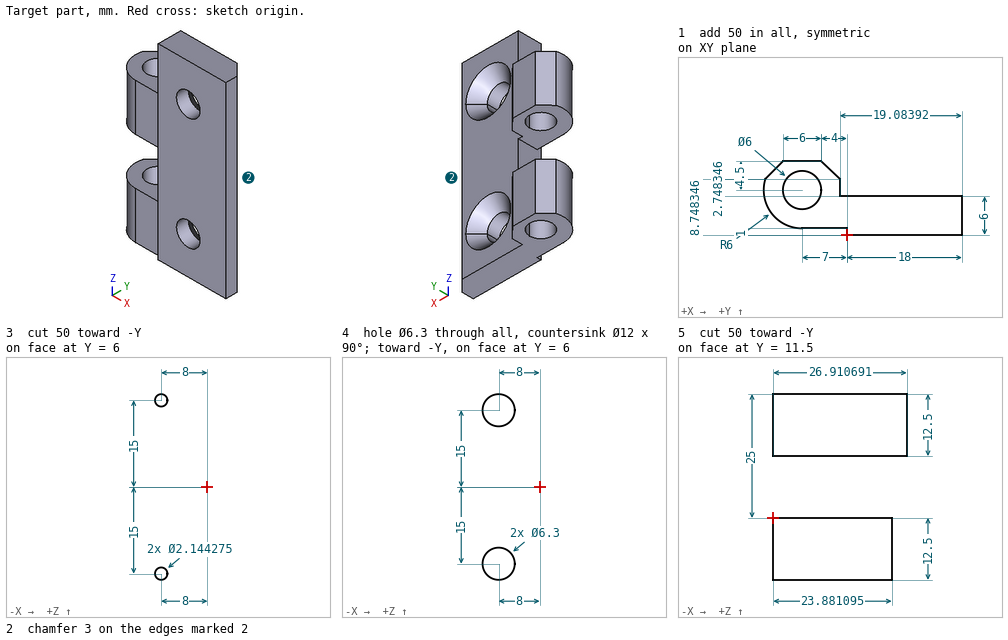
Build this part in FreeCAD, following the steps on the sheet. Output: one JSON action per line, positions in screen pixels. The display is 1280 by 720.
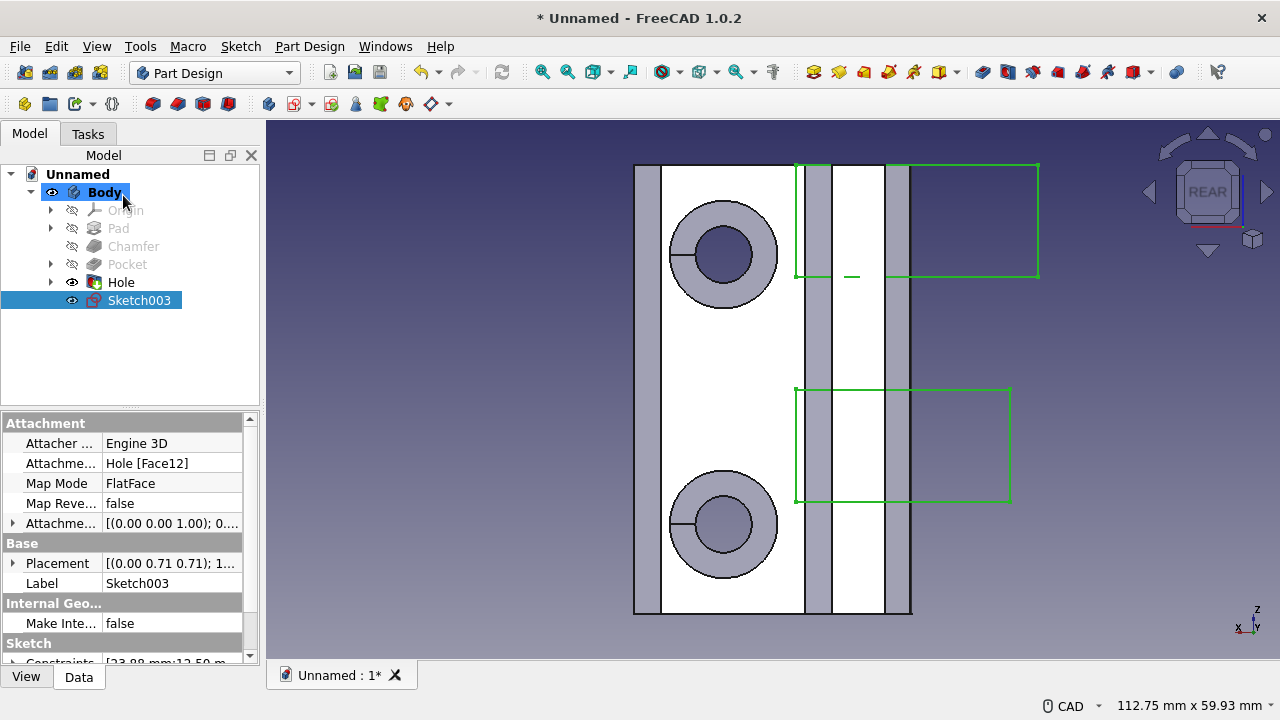
{"action": "left_click", "coordinate": [983, 72]}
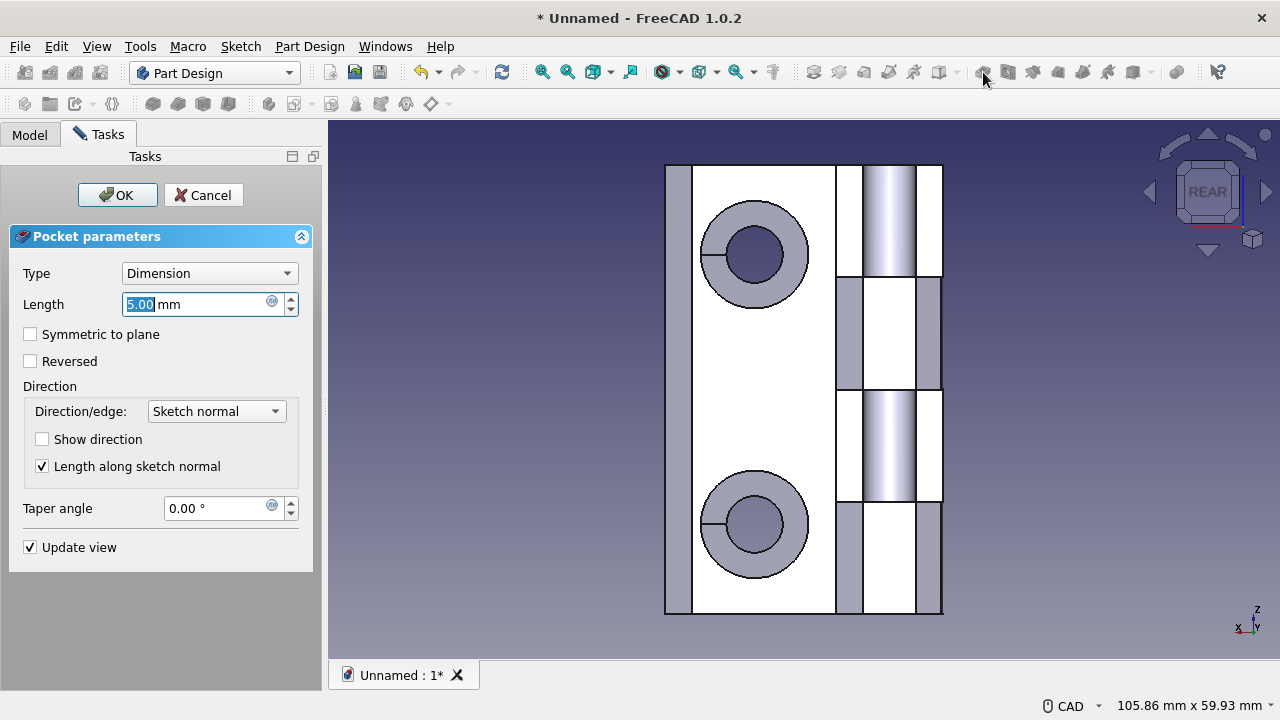
{"action": "type", "text": "50"}
{"action": "key", "text": "Tab"}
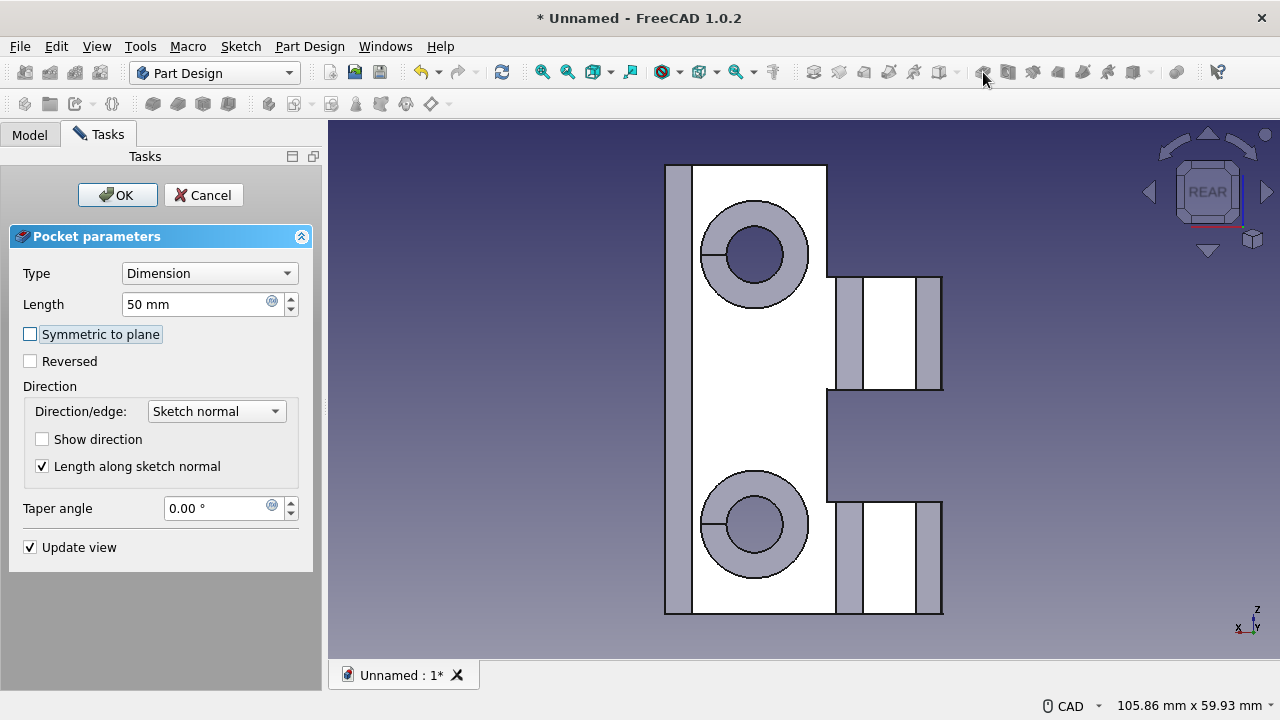
{"action": "left_click", "coordinate": [118, 195]}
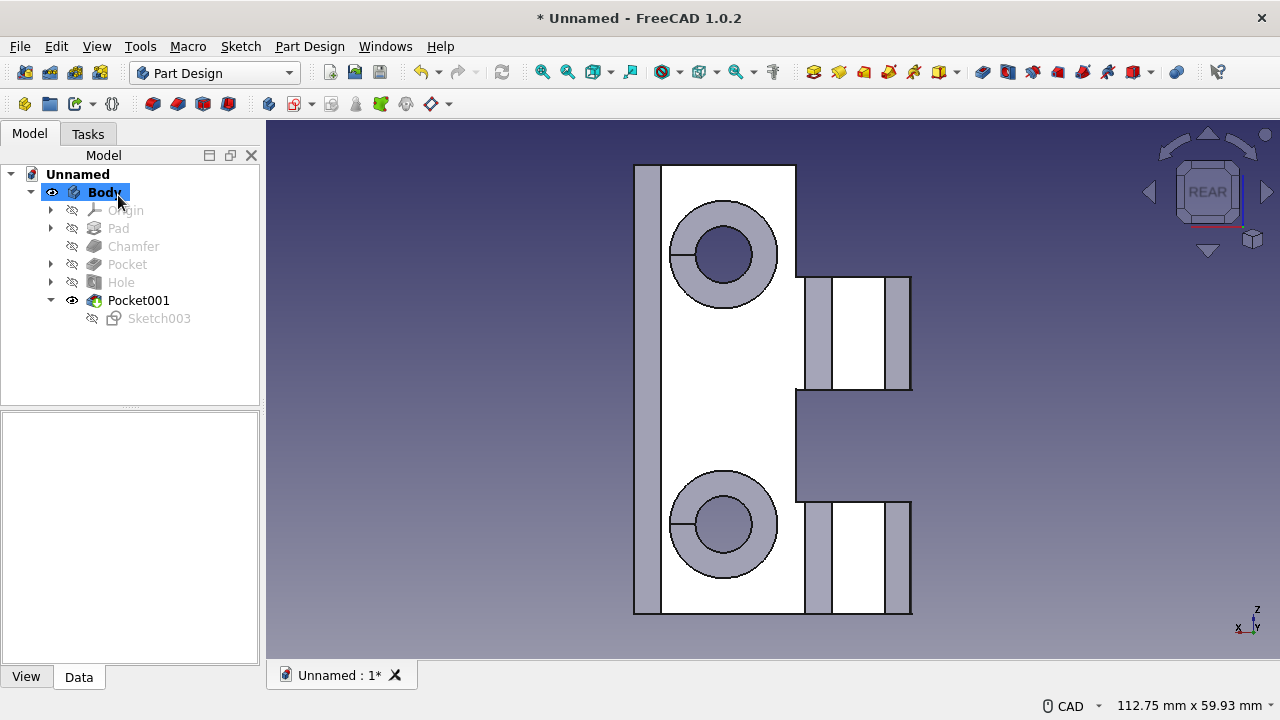
{"action": "key", "text": "0"}